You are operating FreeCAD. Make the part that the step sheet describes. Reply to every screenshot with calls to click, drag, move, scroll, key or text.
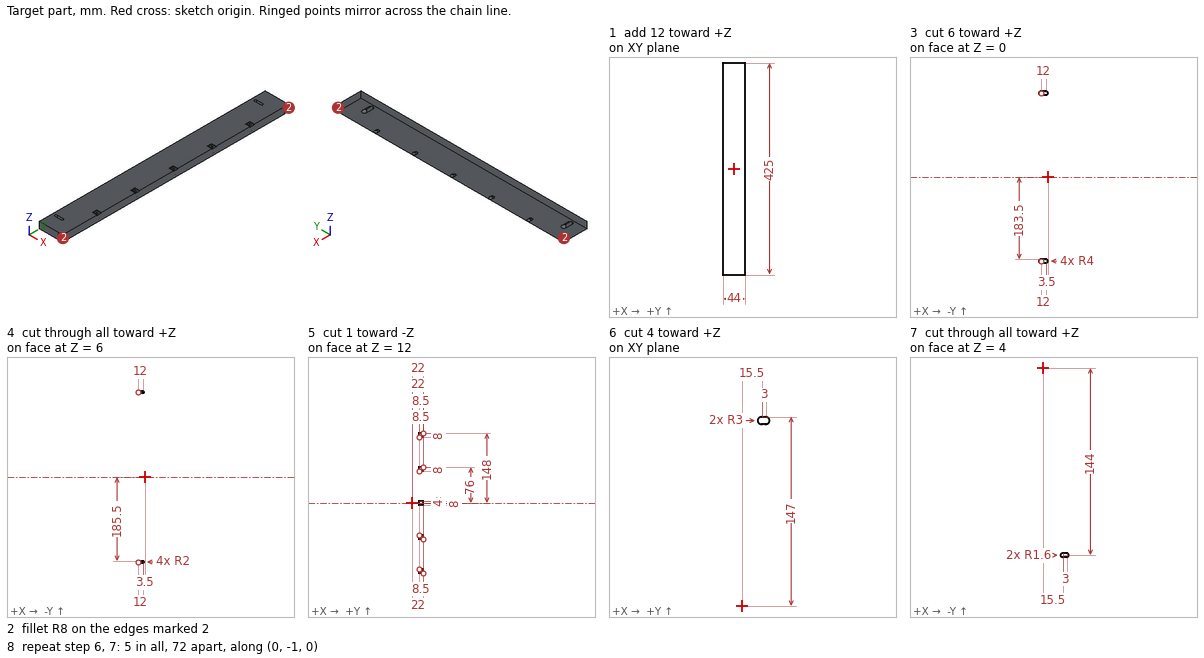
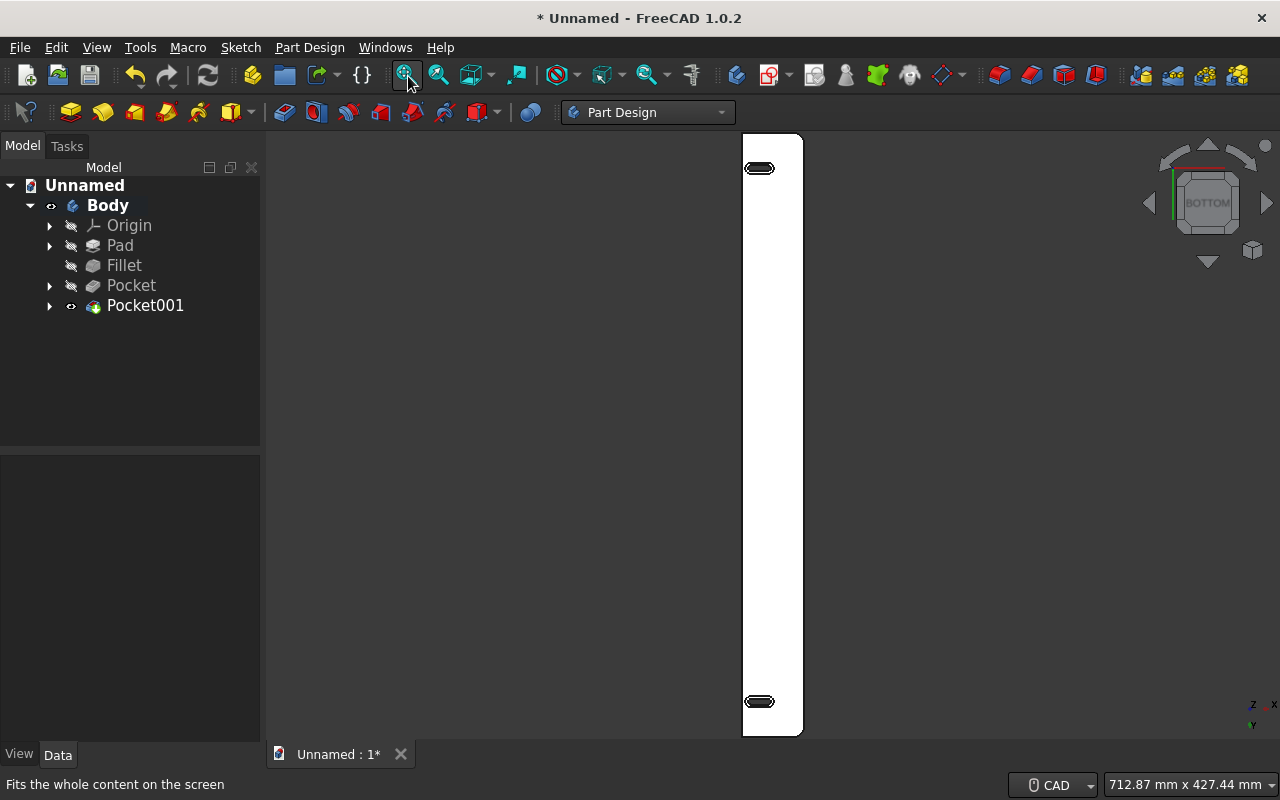
key(0)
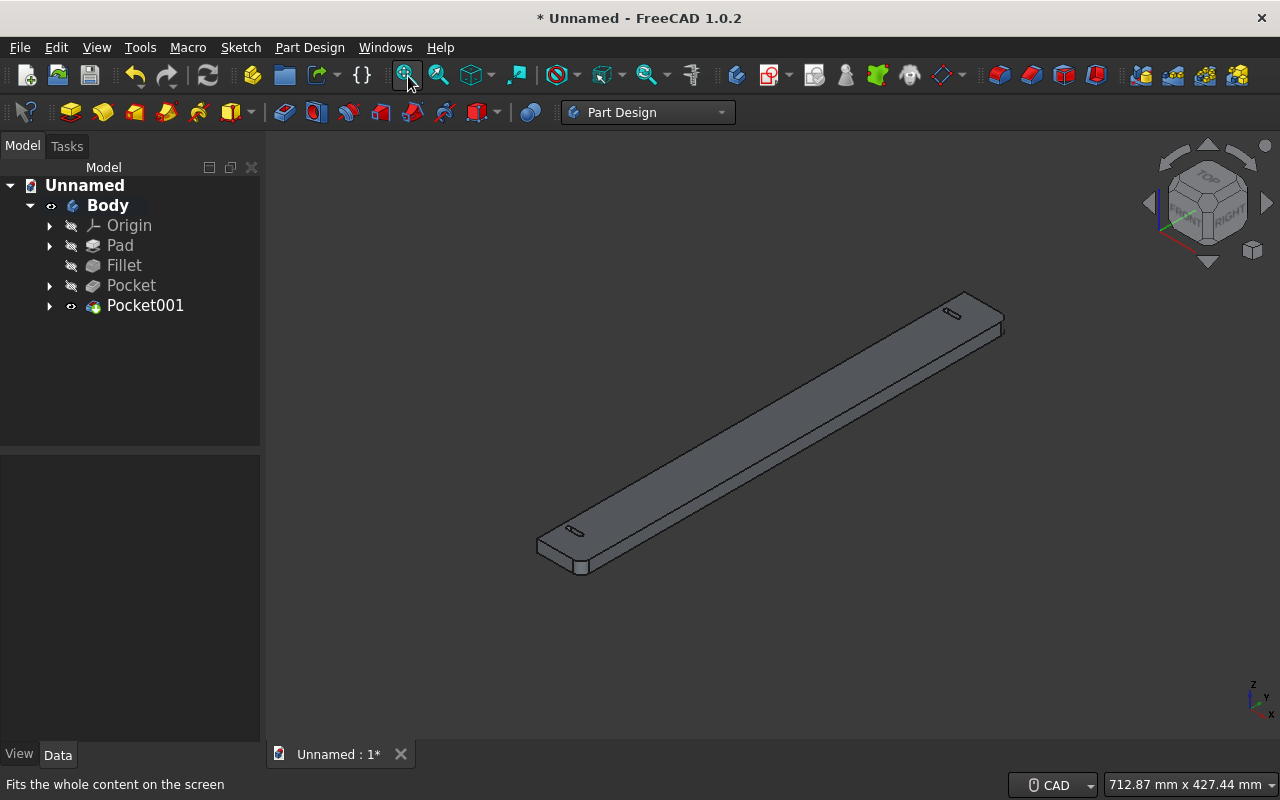
click(895, 357)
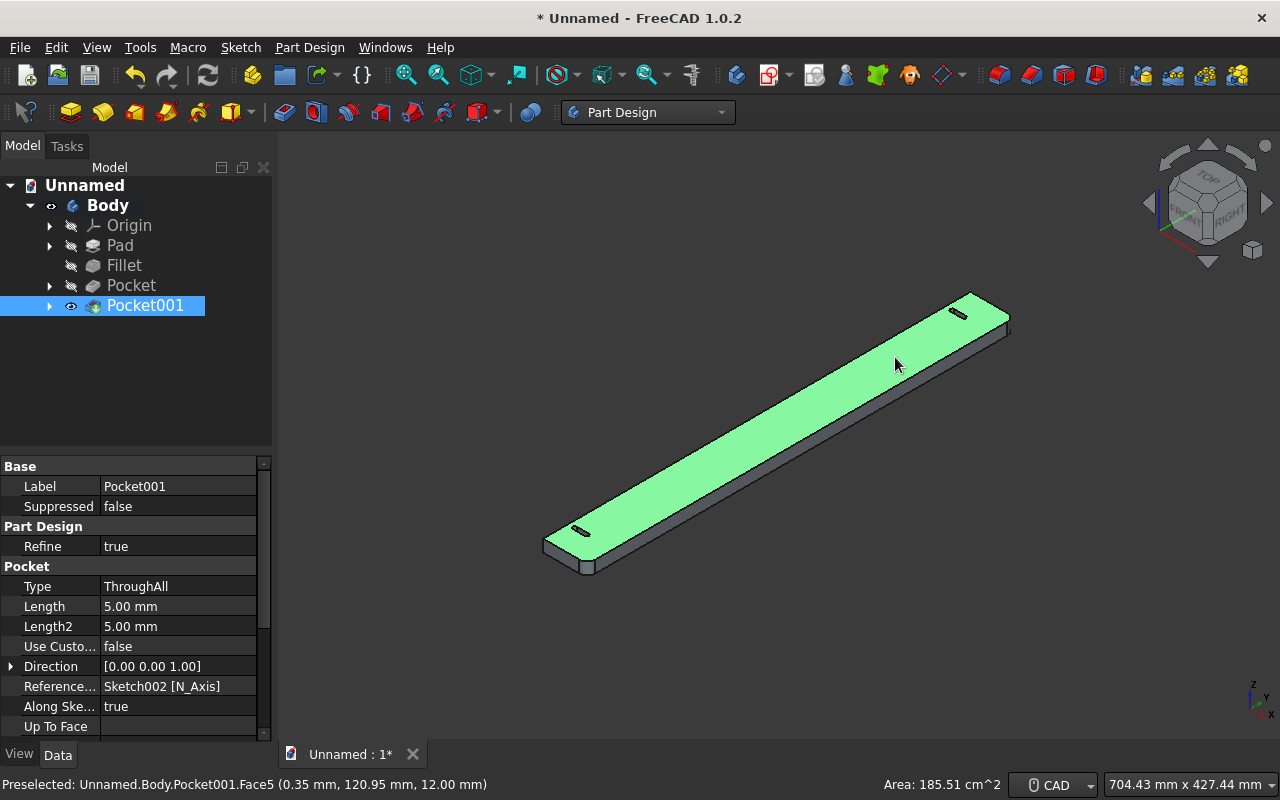
click(770, 76)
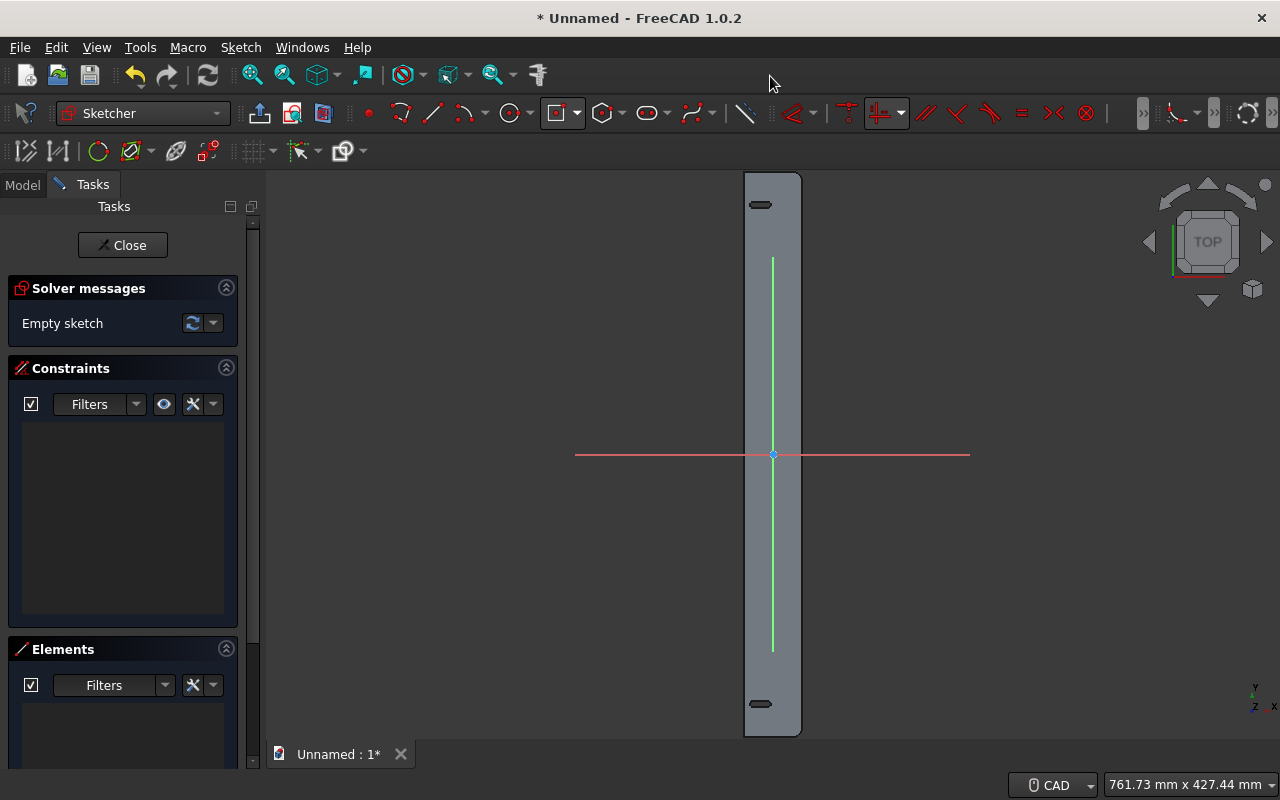
key(g)
key(r)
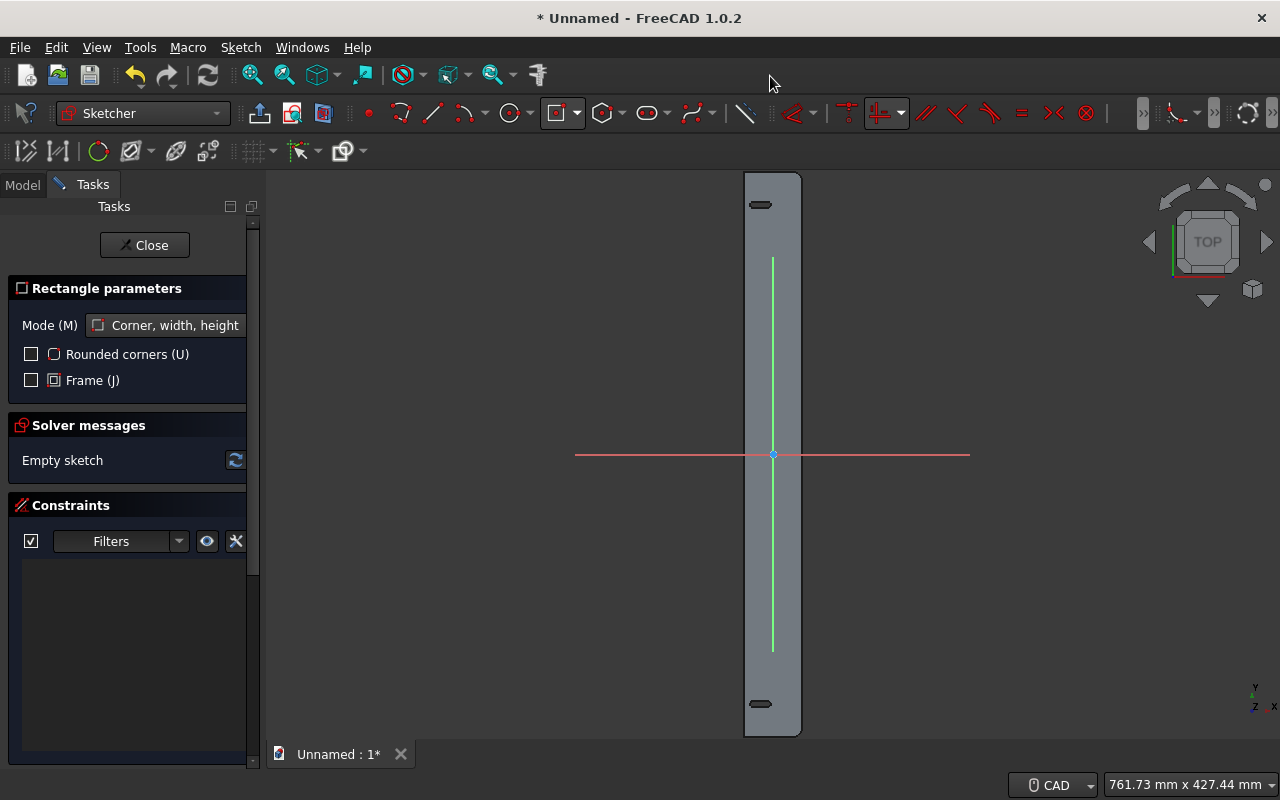
scroll(791, 257, up, 2)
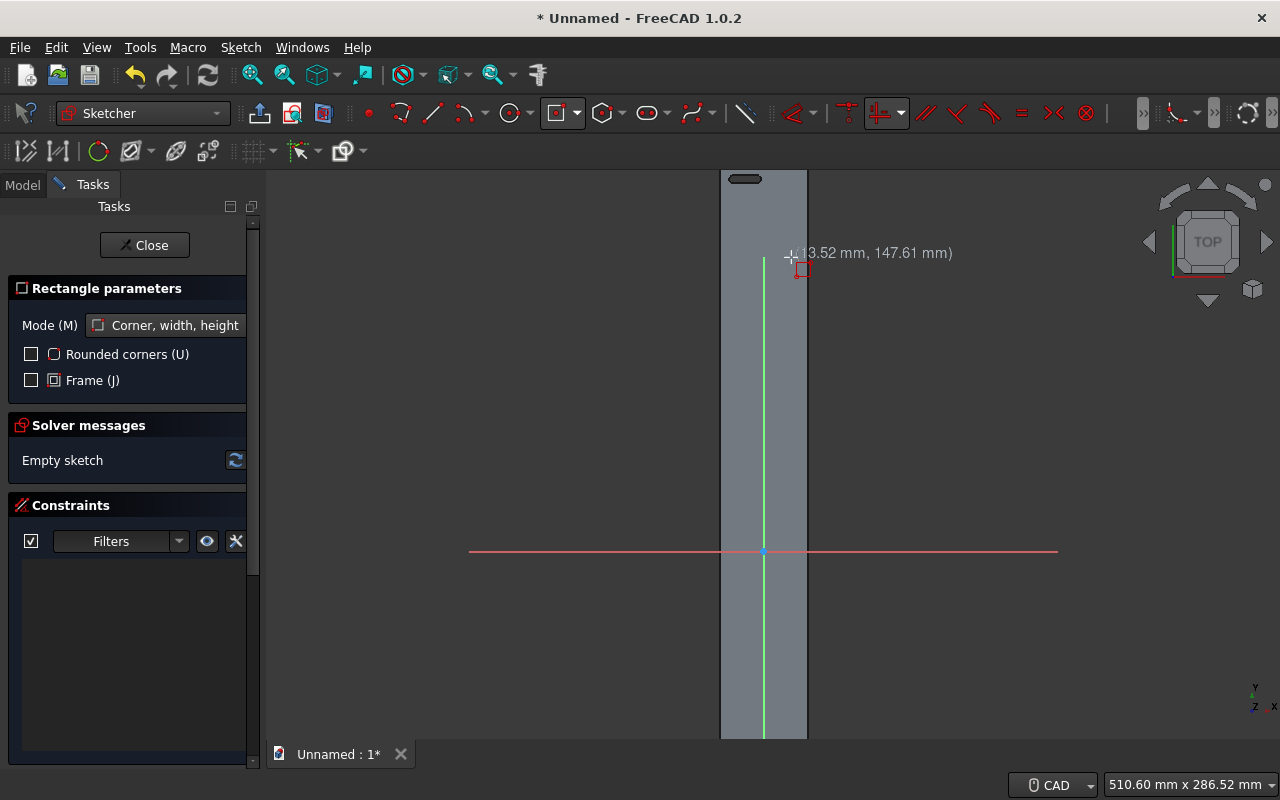
click(791, 258)
click(808, 274)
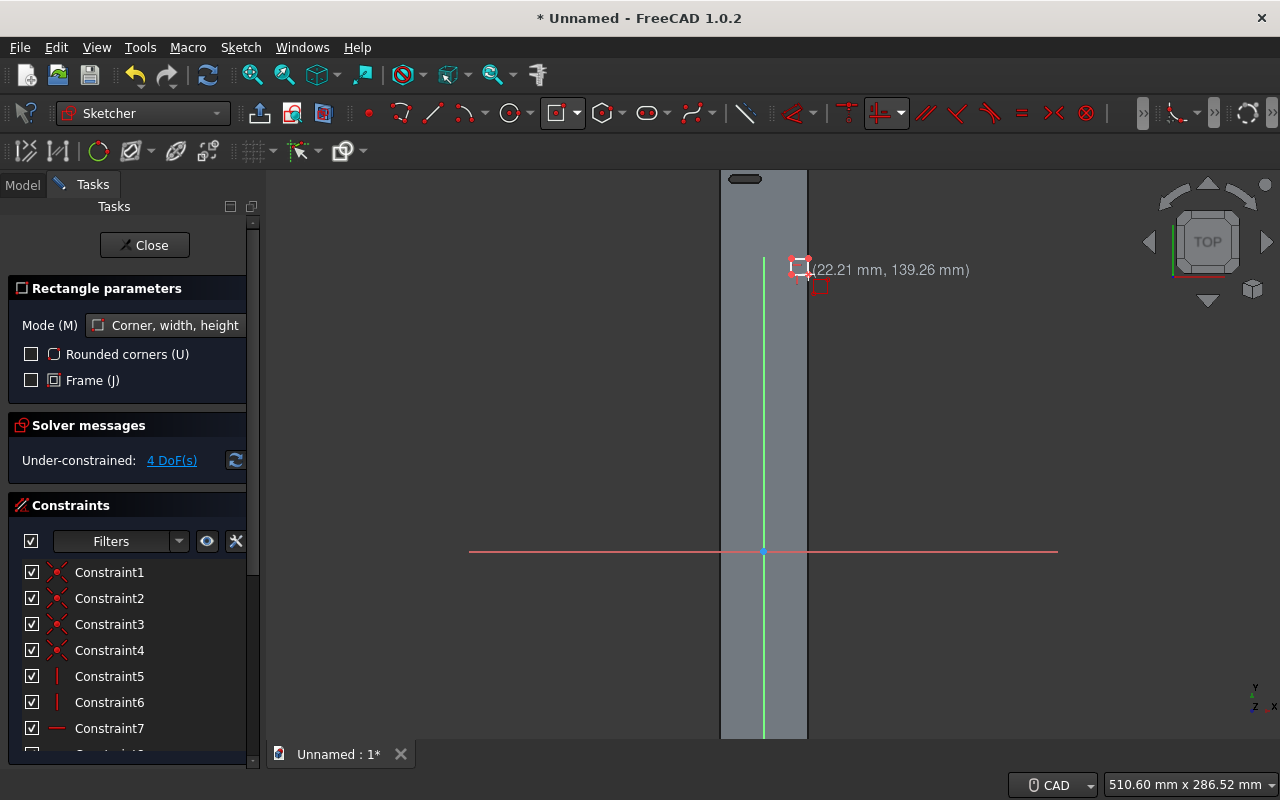
click(791, 401)
click(808, 417)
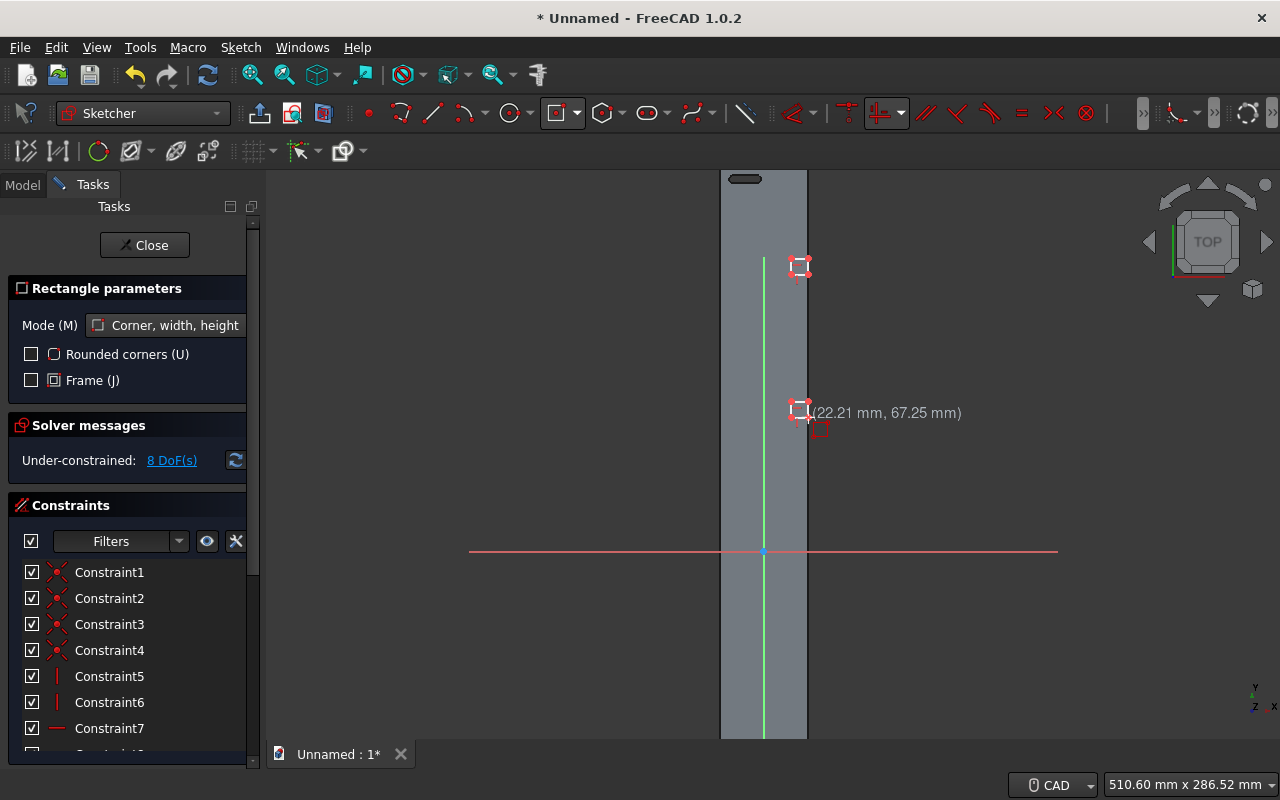
scroll(791, 544, up, 4)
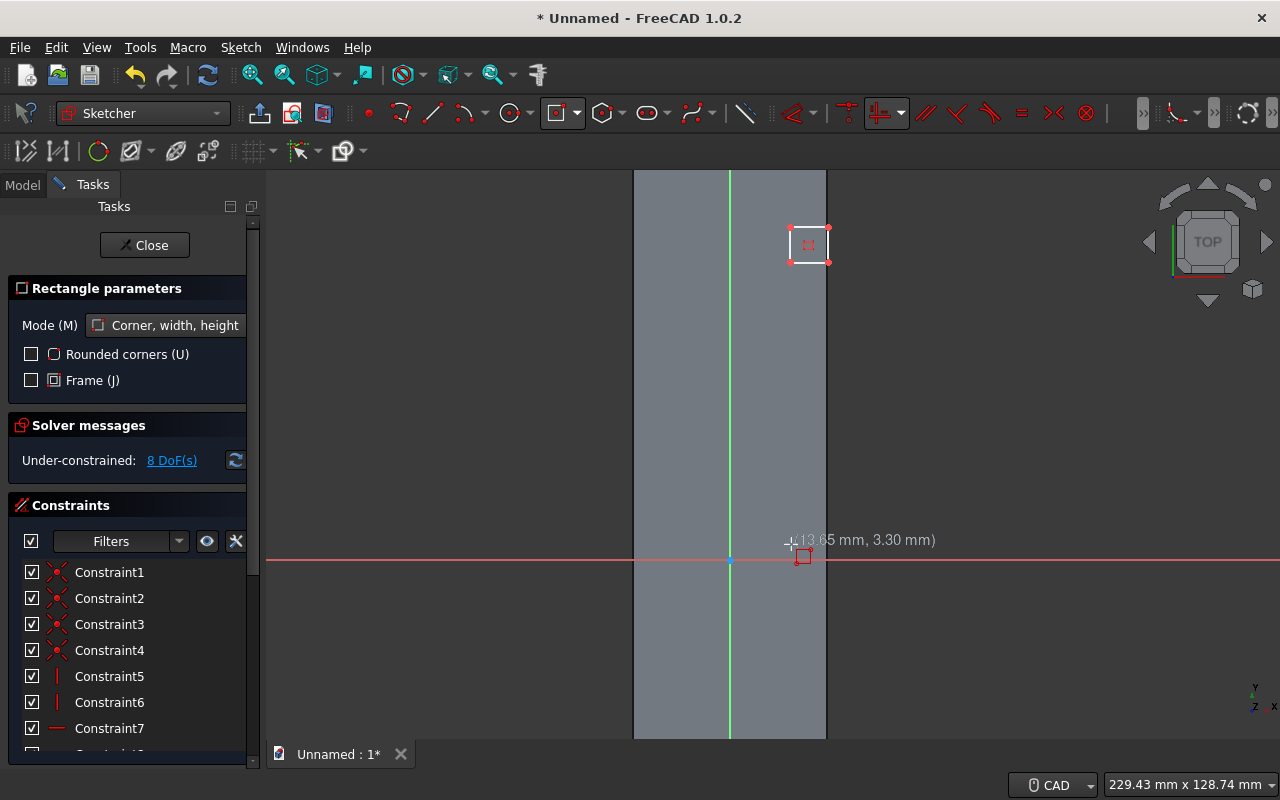
click(790, 542)
click(827, 578)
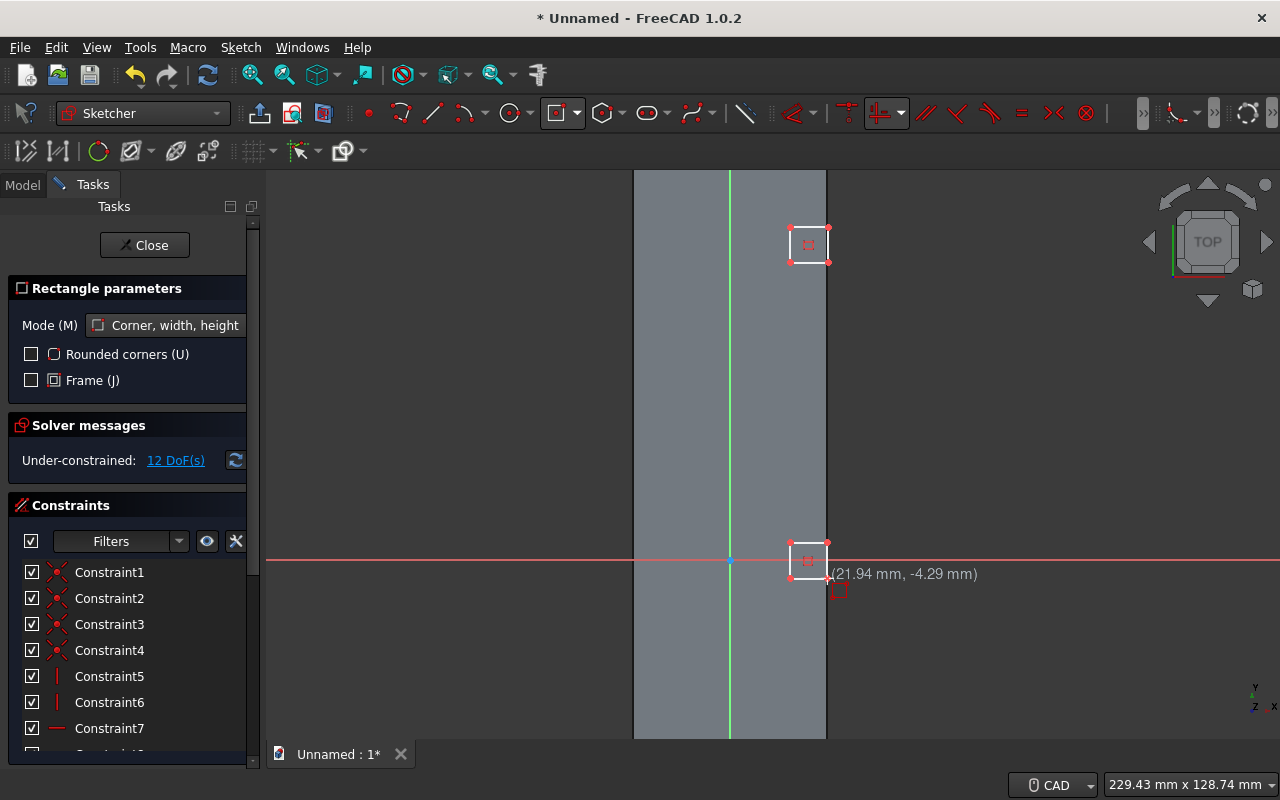
scroll(673, 409, down, 6)